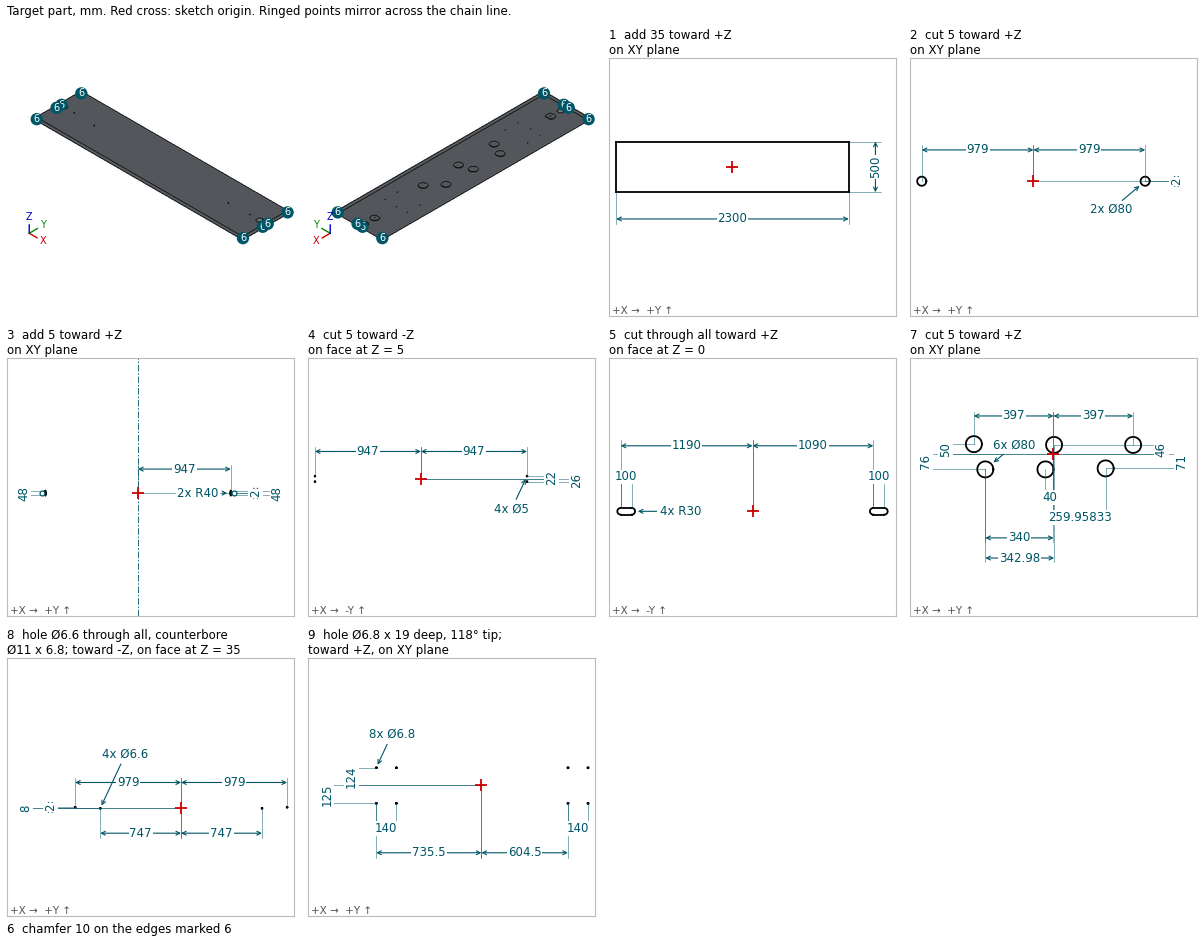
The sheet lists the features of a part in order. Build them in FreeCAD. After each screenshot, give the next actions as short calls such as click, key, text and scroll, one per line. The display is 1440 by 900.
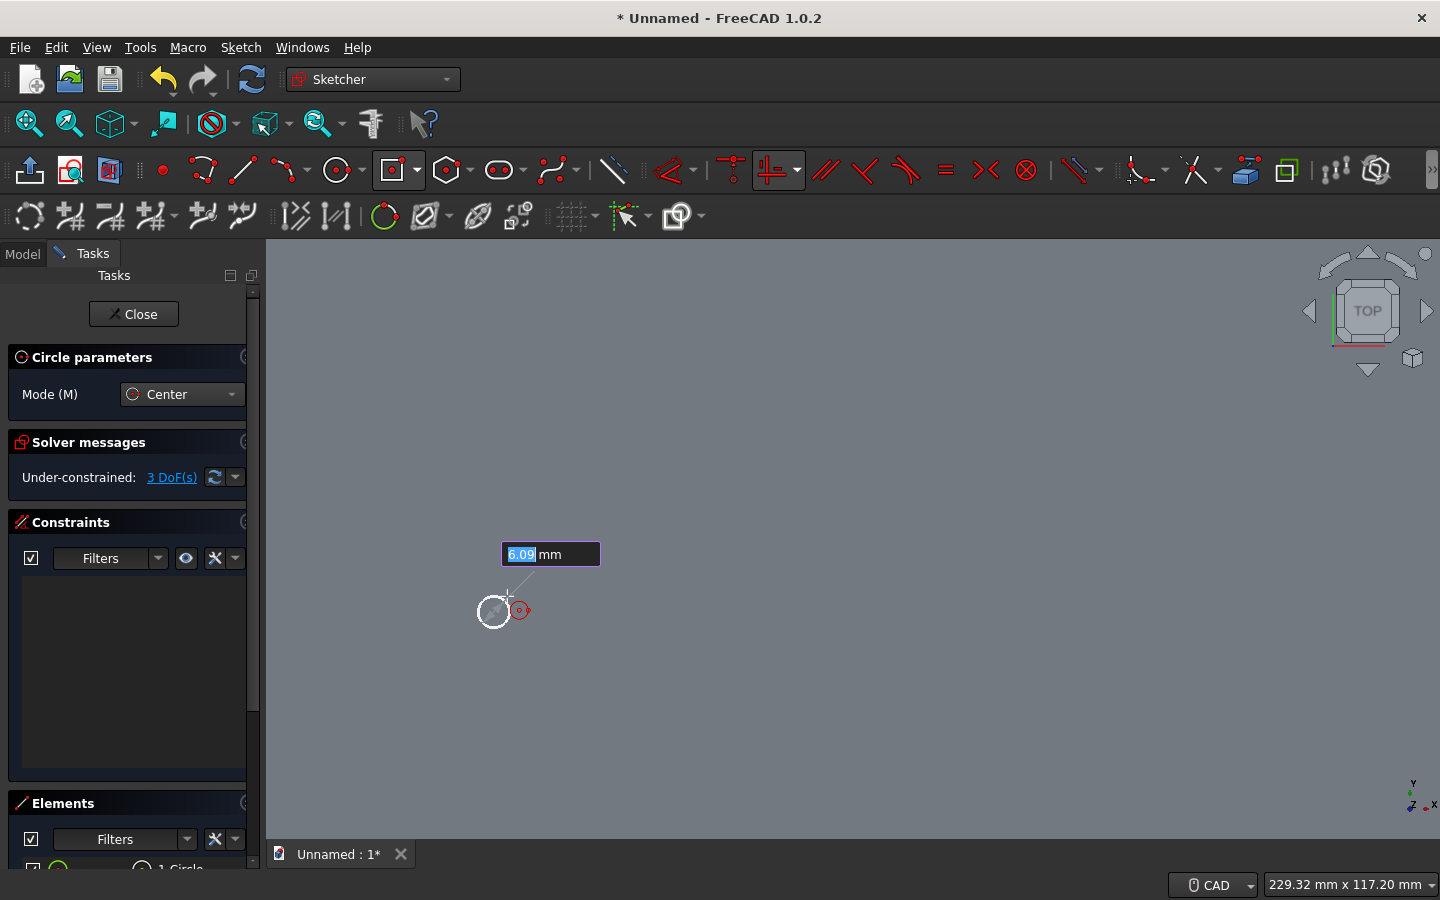
click(503, 592)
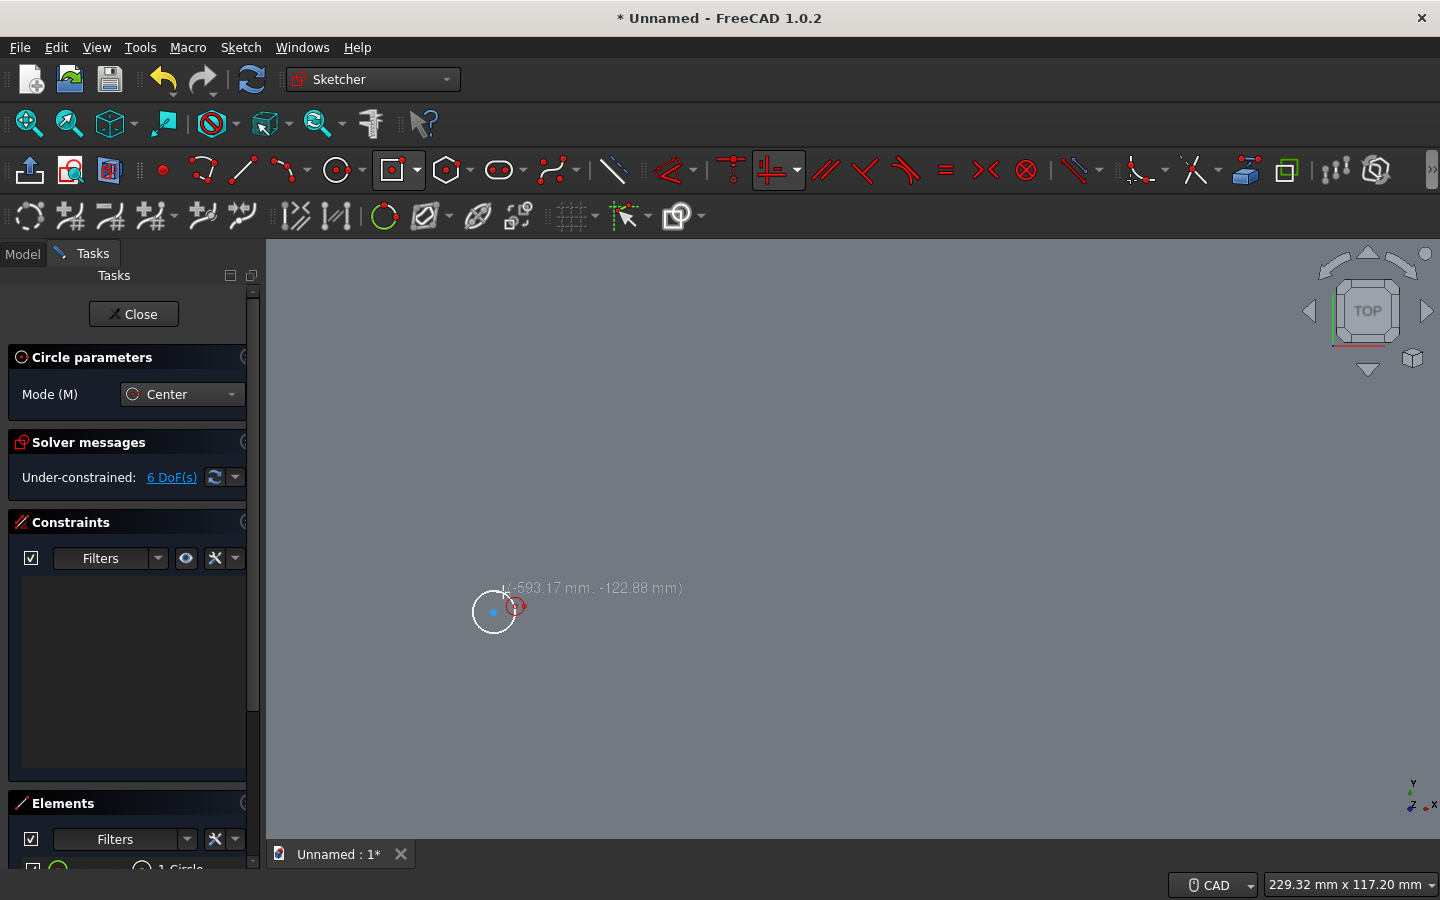
scroll(507, 596, down, 12)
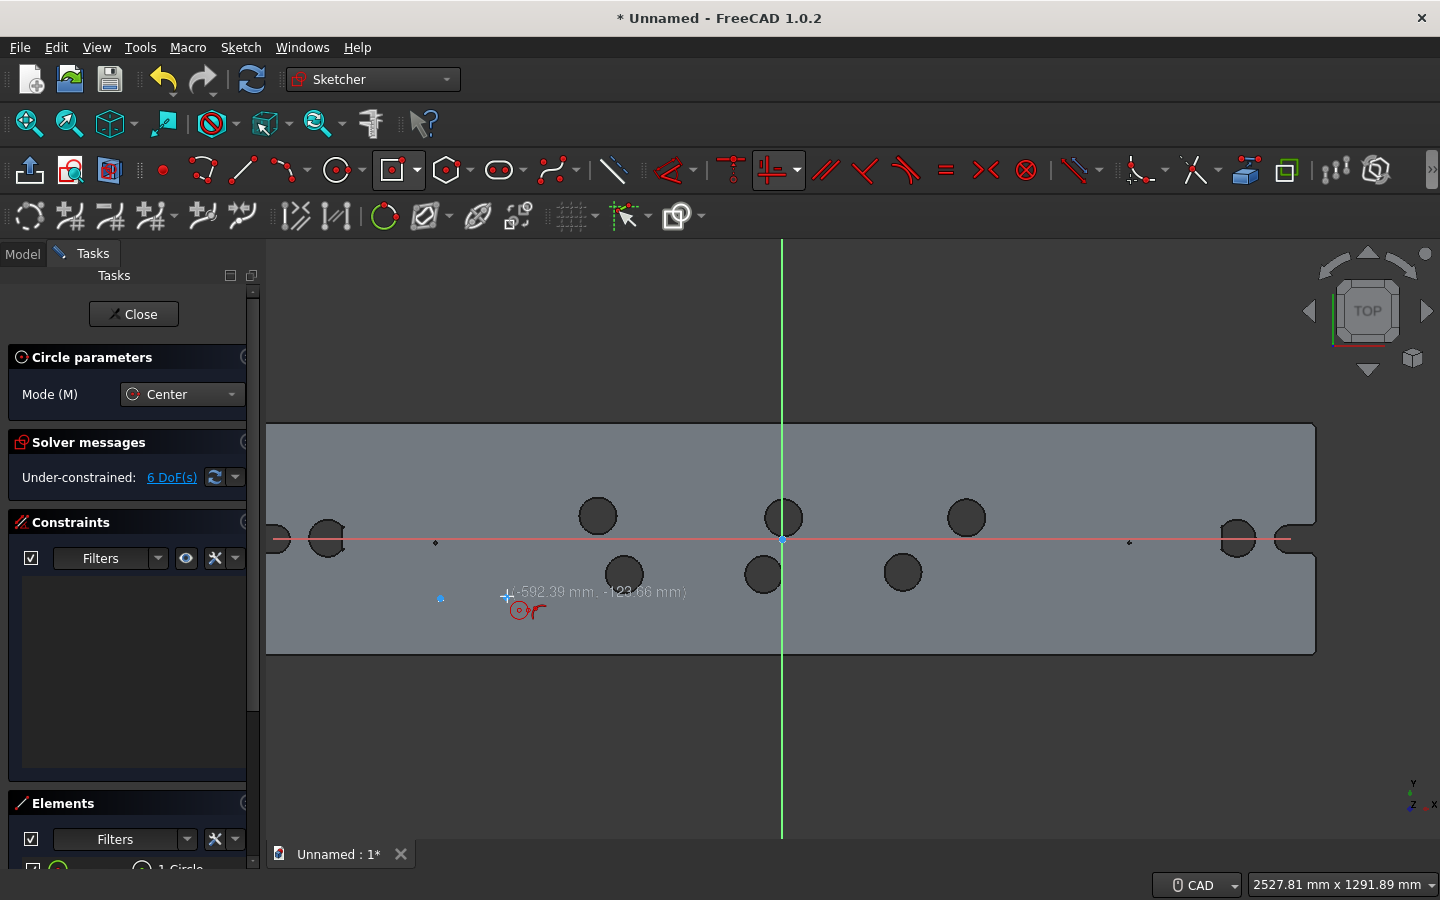
scroll(441, 482, up, 14)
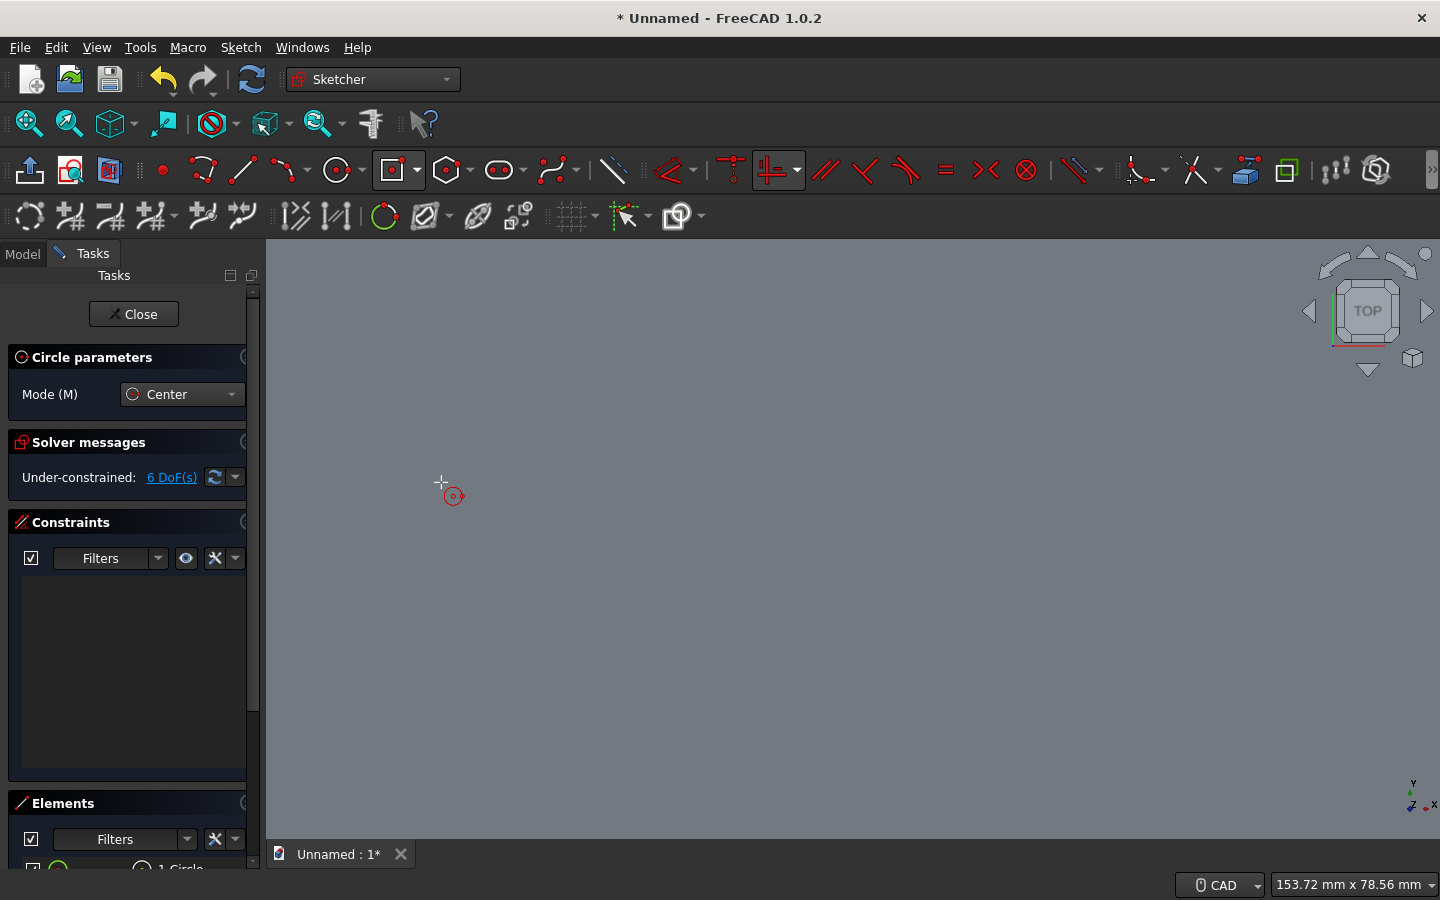
scroll(441, 482, down, 14)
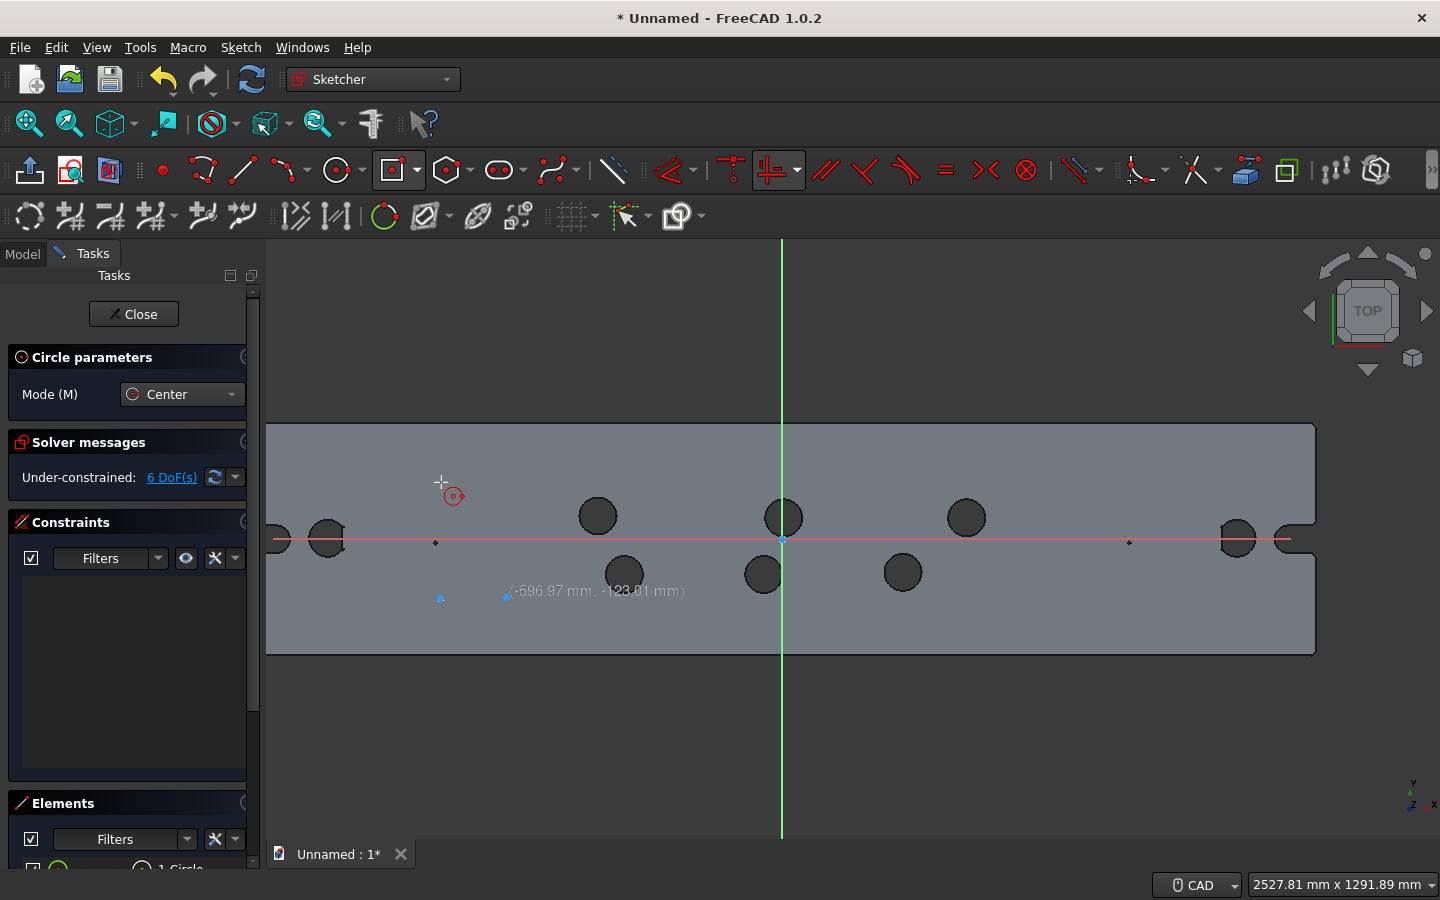
click(441, 482)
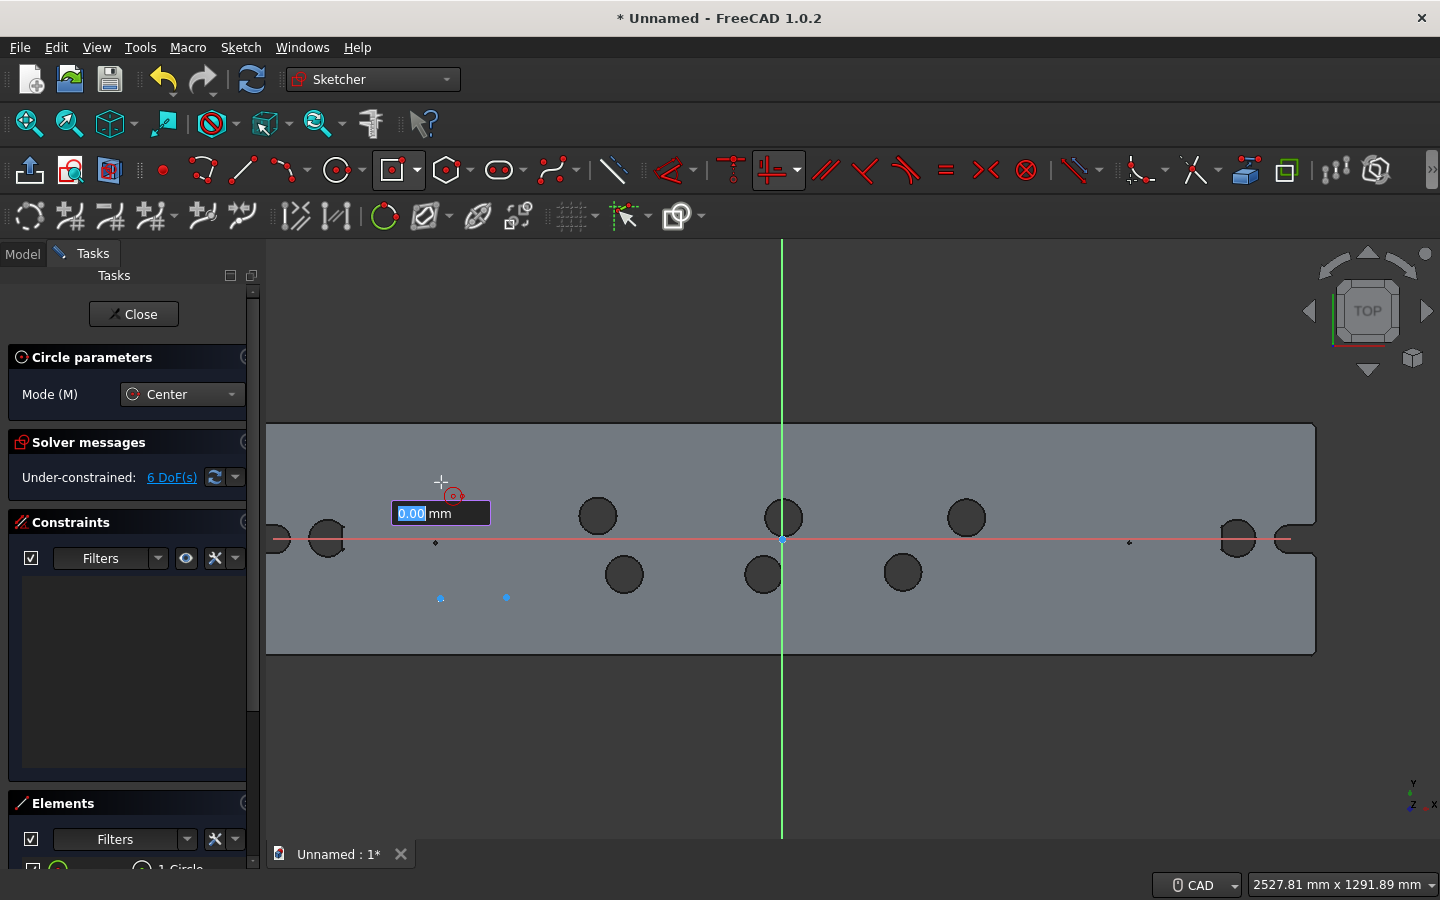
scroll(442, 480, up, 12)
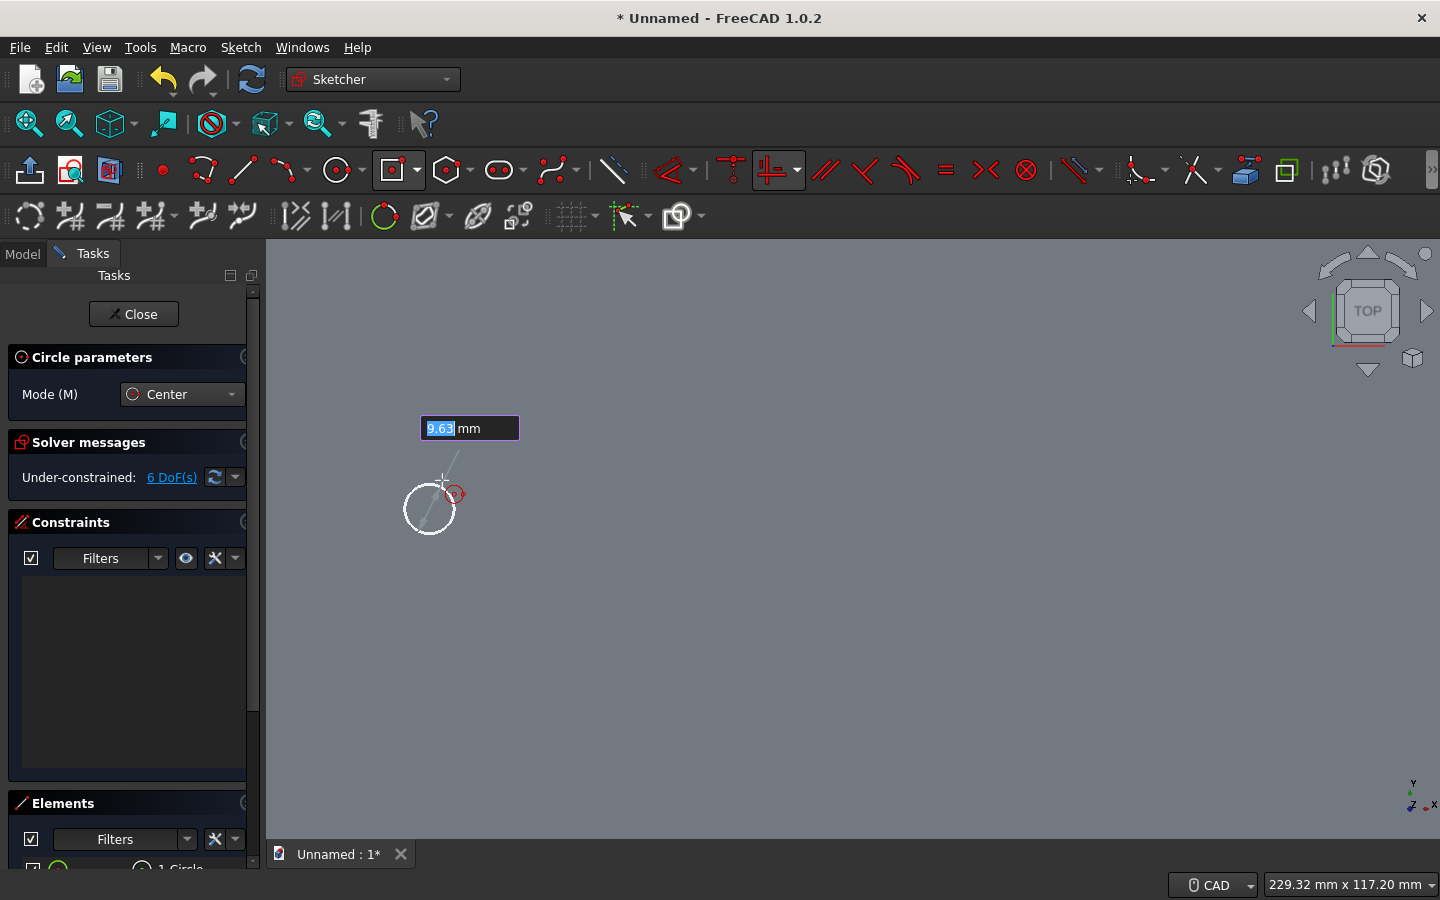
click(439, 481)